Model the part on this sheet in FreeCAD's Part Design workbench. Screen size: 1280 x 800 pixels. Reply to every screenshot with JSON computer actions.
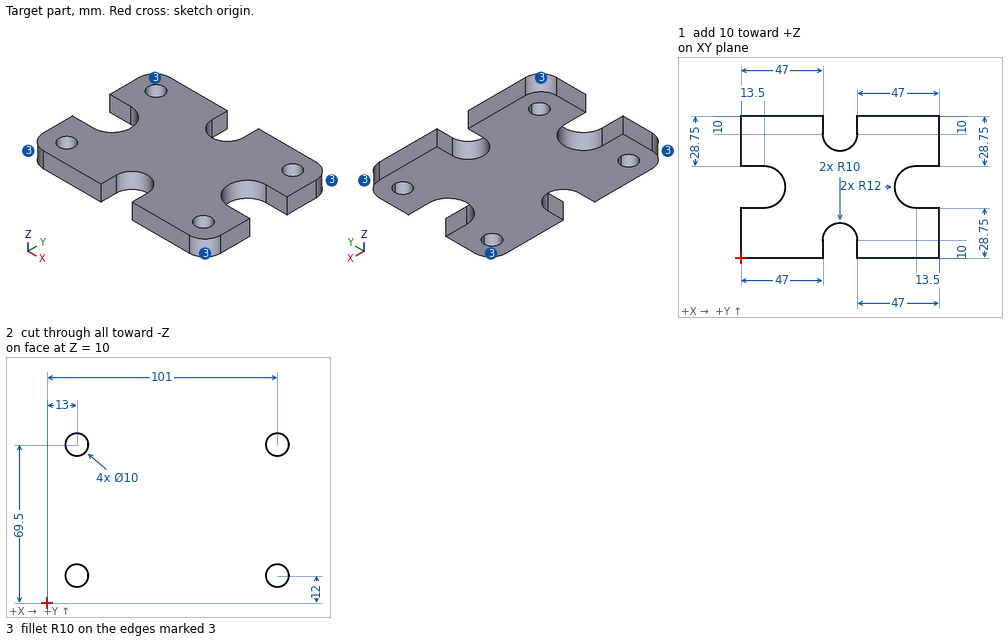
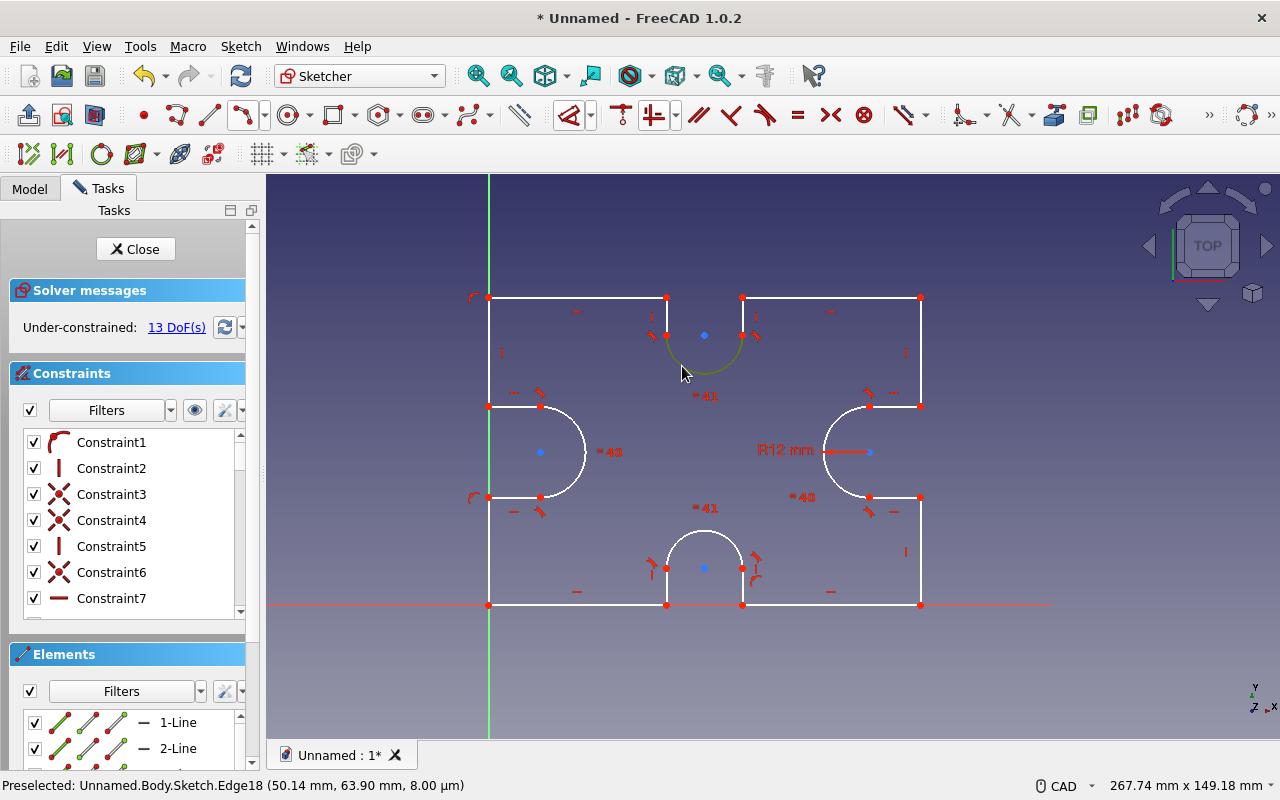
{"action": "key", "text": "k r"}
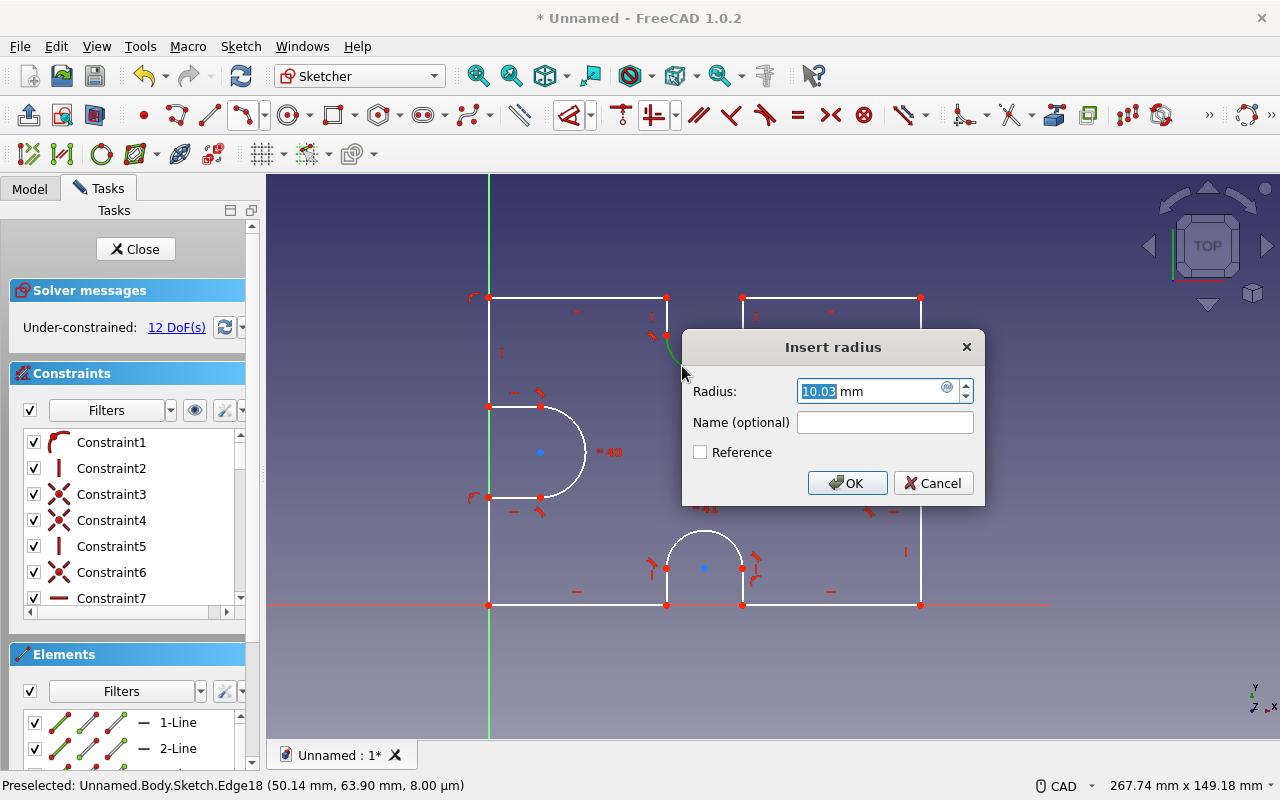
{"action": "type", "text": "10"}
{"action": "key", "text": "Return"}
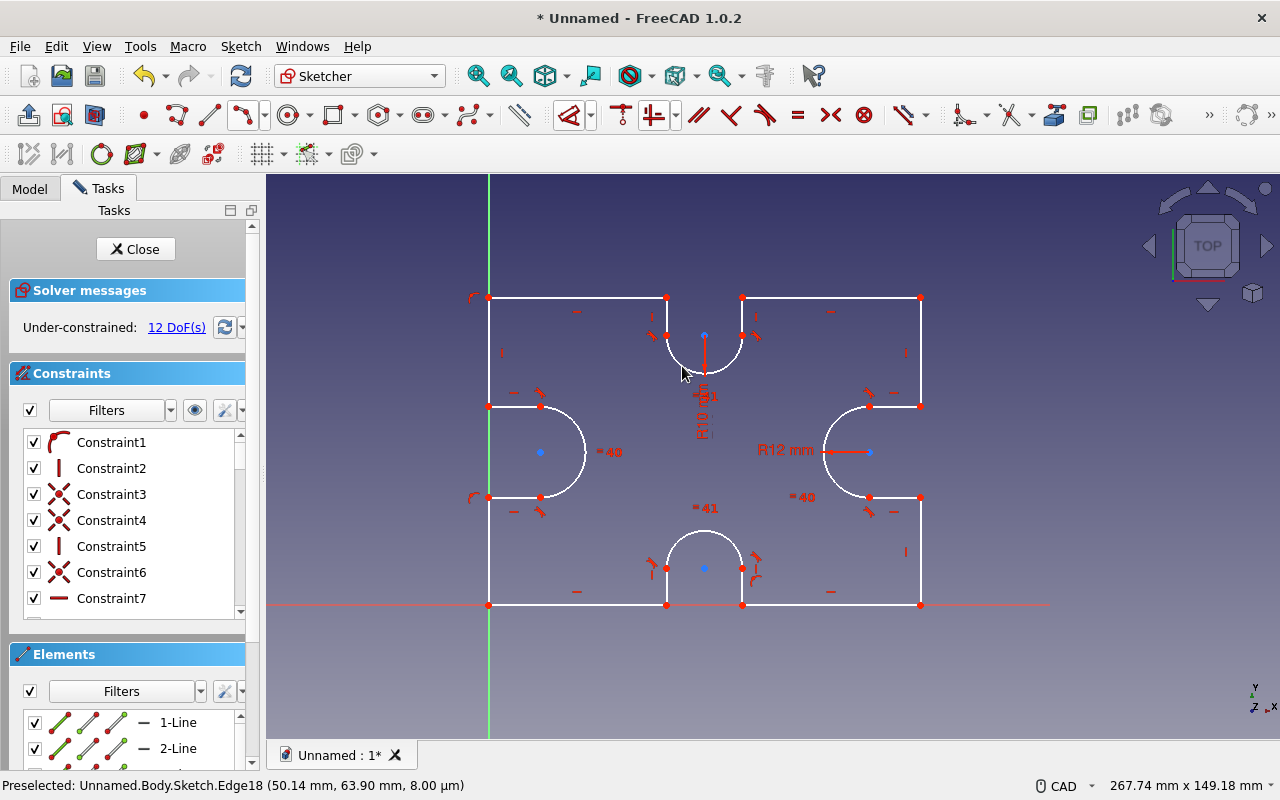
{"action": "scroll", "coordinate": [742, 580], "scroll_direction": "up", "scroll_amount": 2}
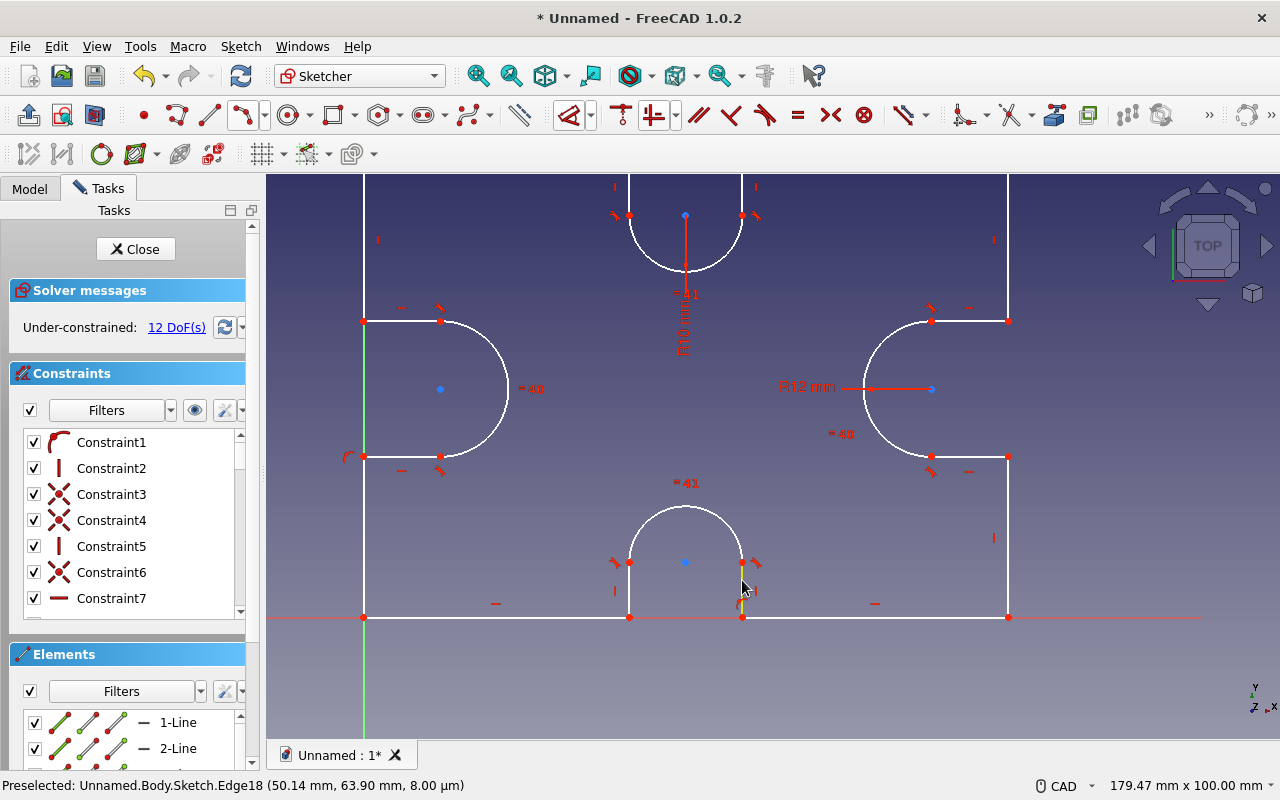
{"action": "left_click", "coordinate": [742, 579]}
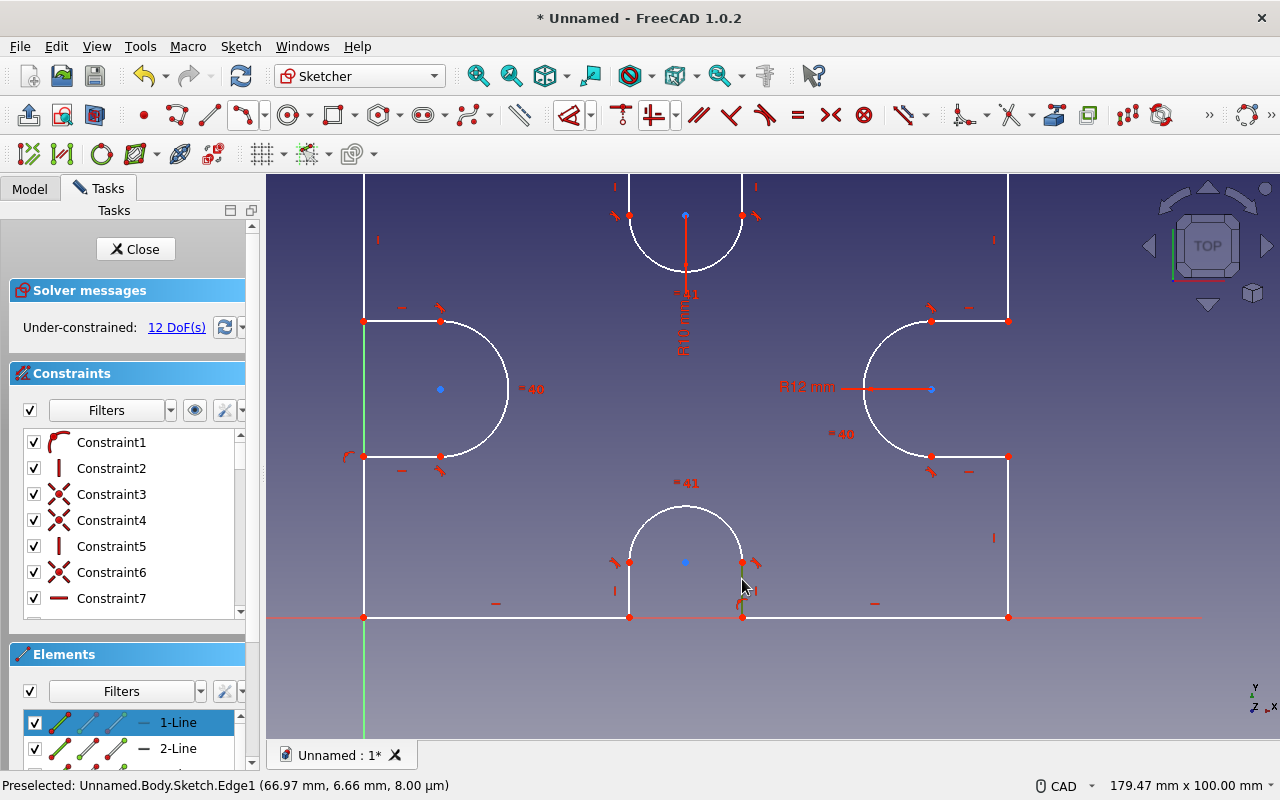
{"action": "left_click", "coordinate": [590, 116]}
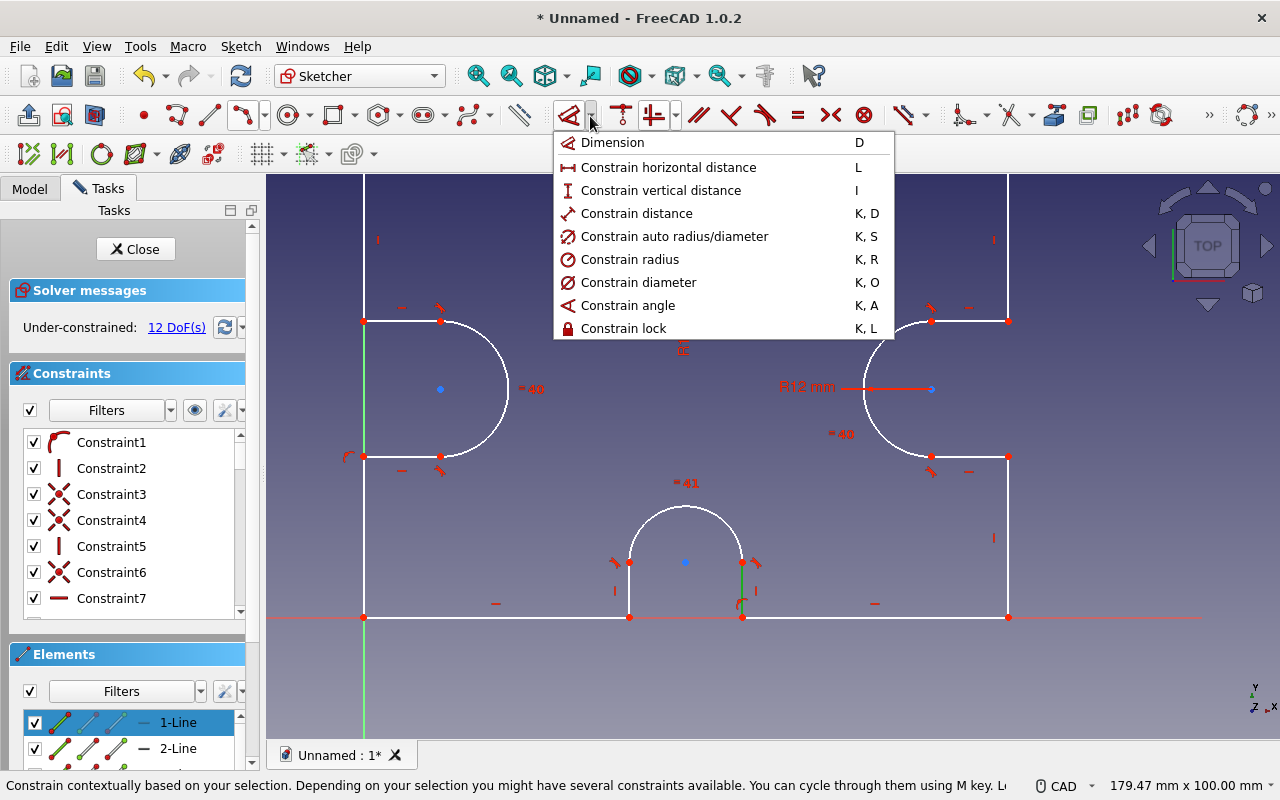
{"action": "left_click", "coordinate": [724, 190]}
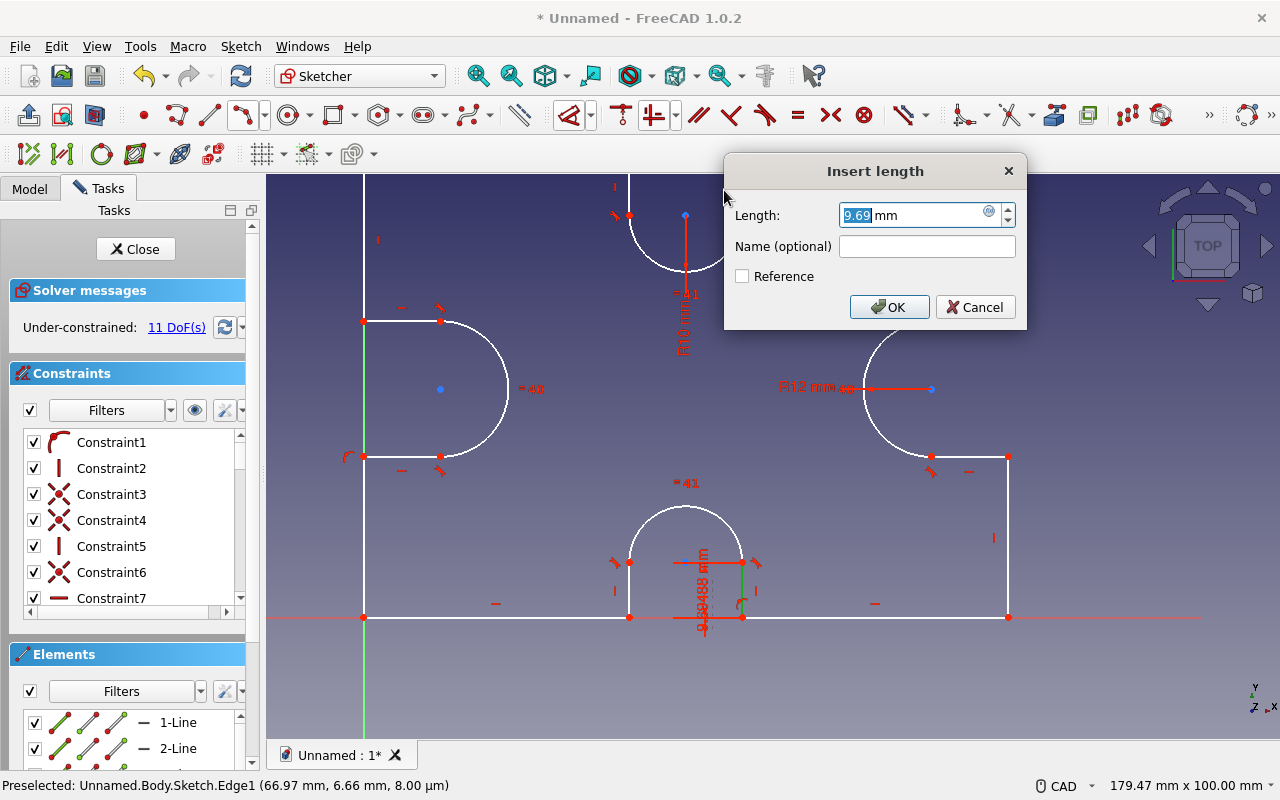
{"action": "type", "text": "10"}
{"action": "key", "text": "Return"}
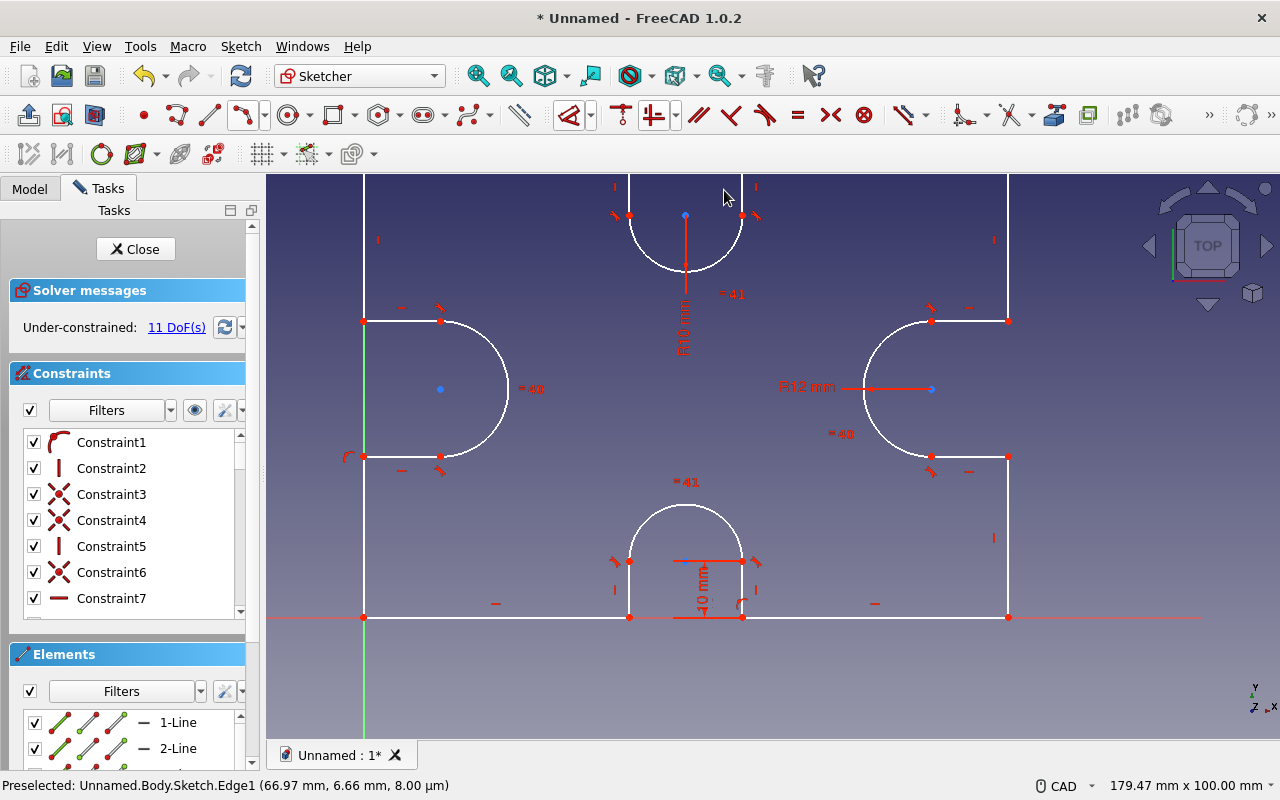
{"action": "left_click", "coordinate": [822, 618]}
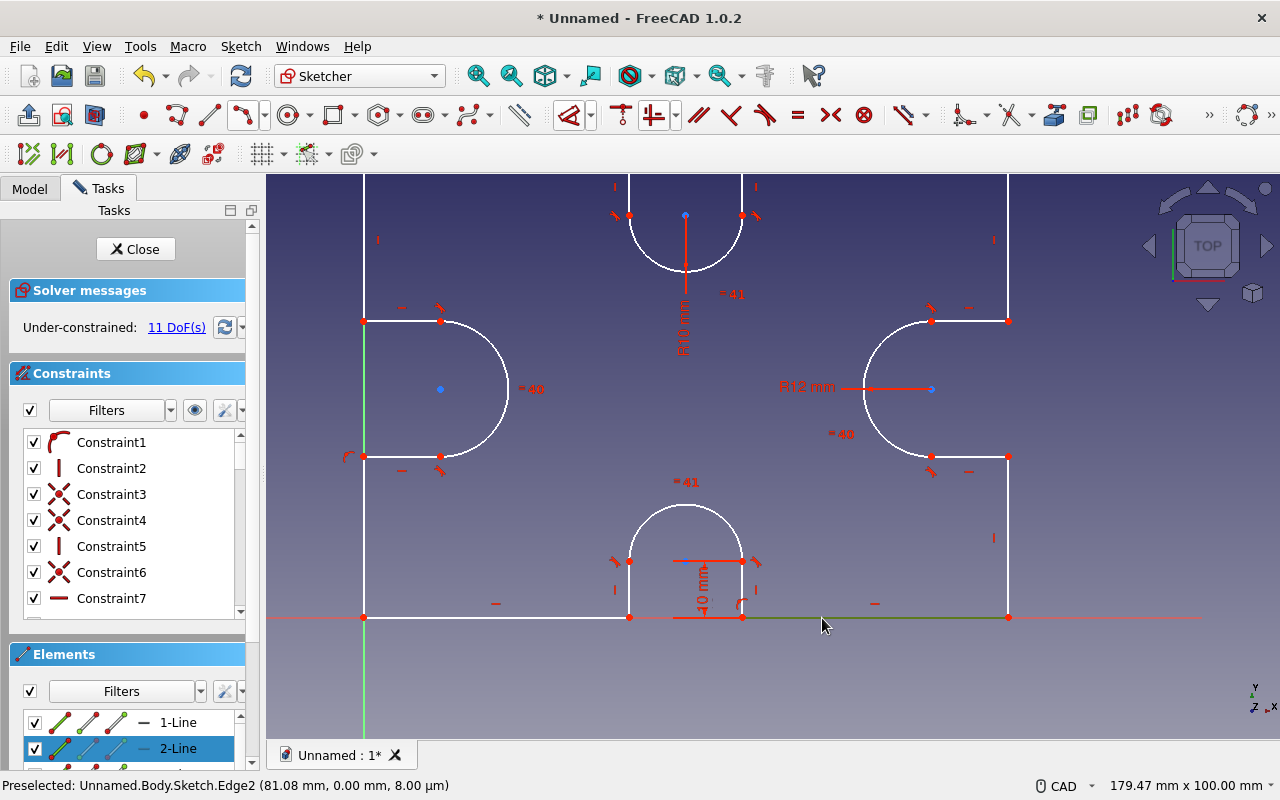
{"action": "left_click", "coordinate": [590, 116]}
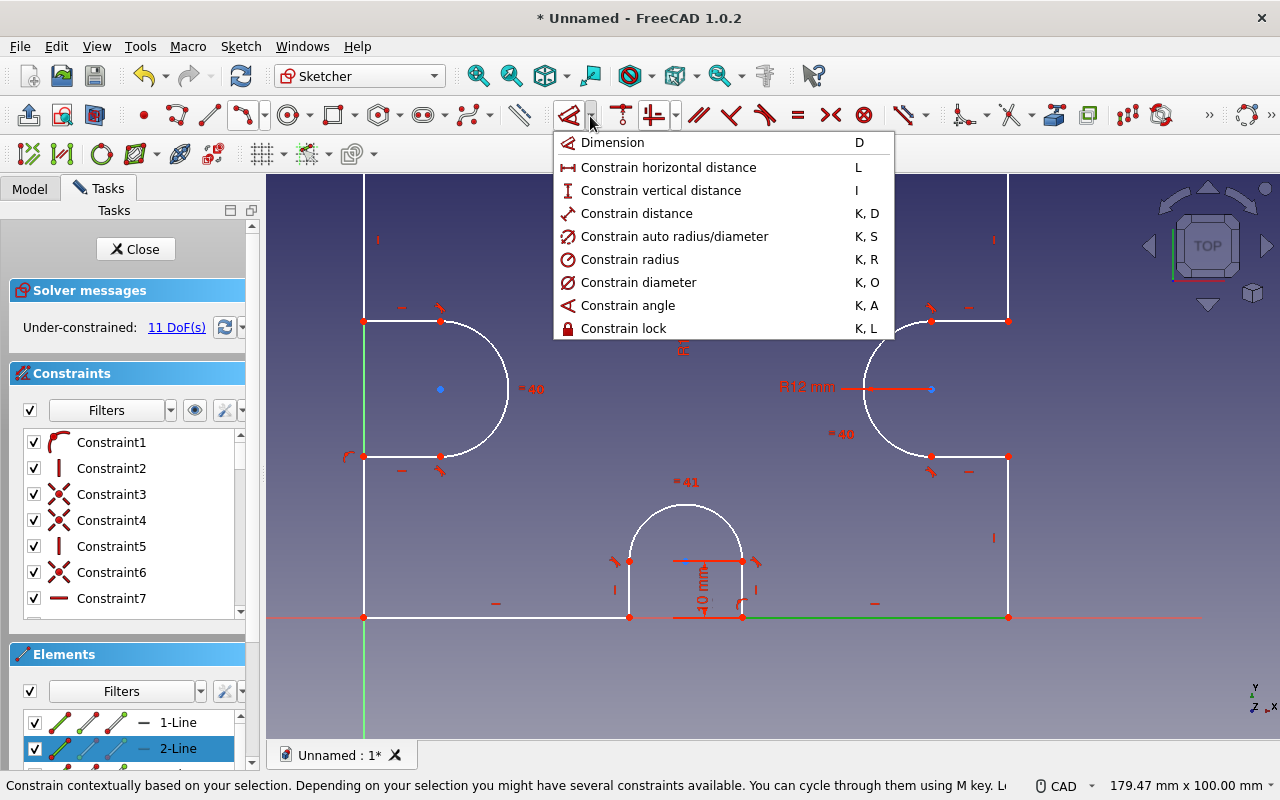
{"action": "left_click", "coordinate": [724, 168]}